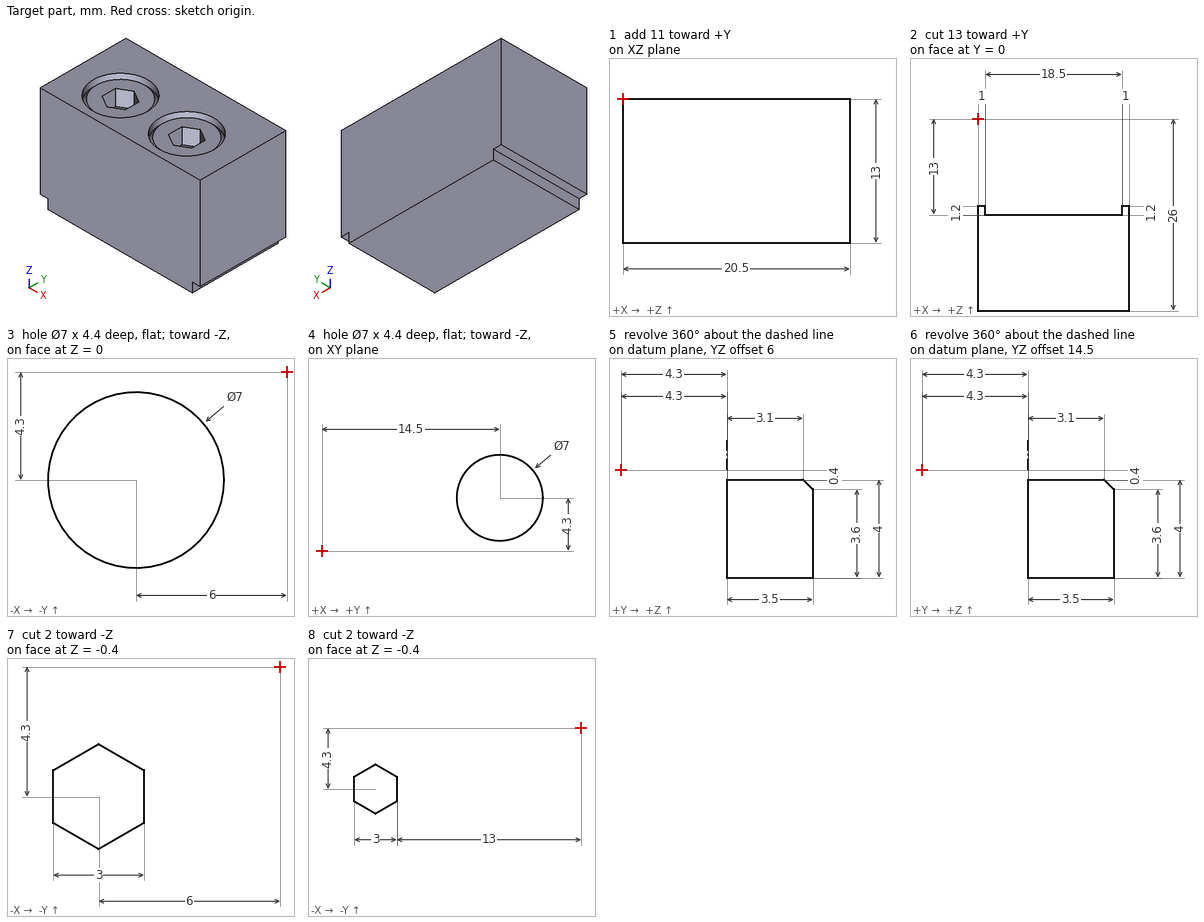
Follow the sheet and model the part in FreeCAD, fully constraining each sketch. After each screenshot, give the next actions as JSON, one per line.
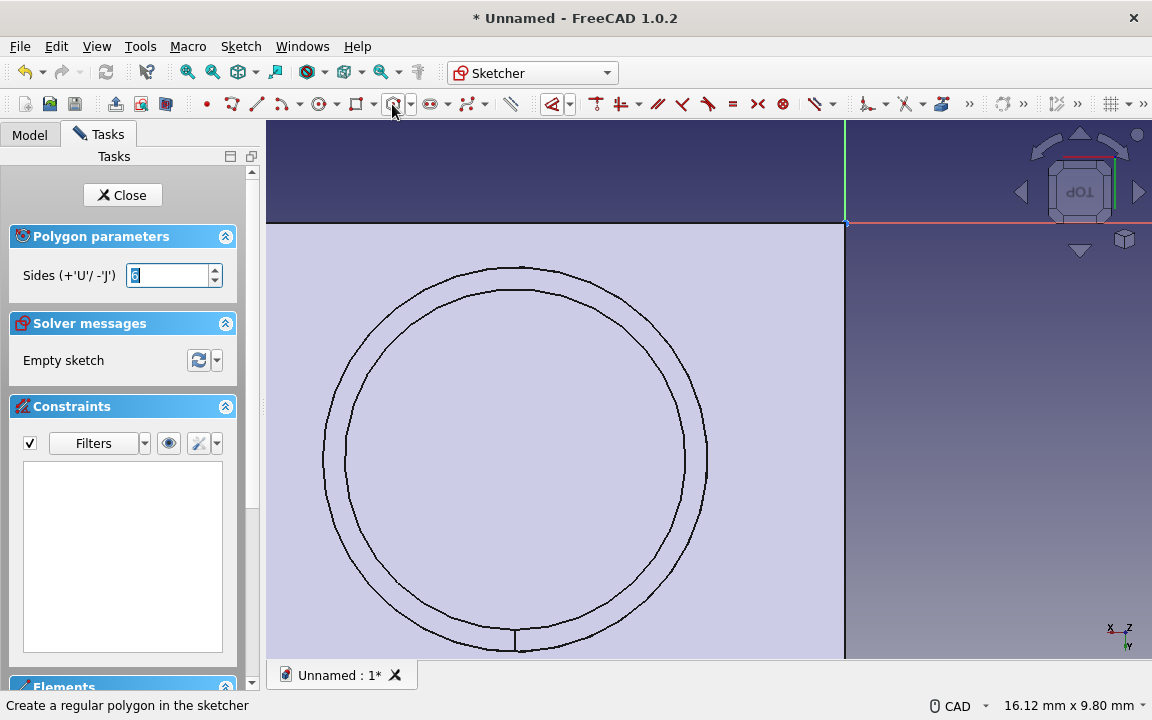
{"action": "left_click", "coordinate": [515, 460]}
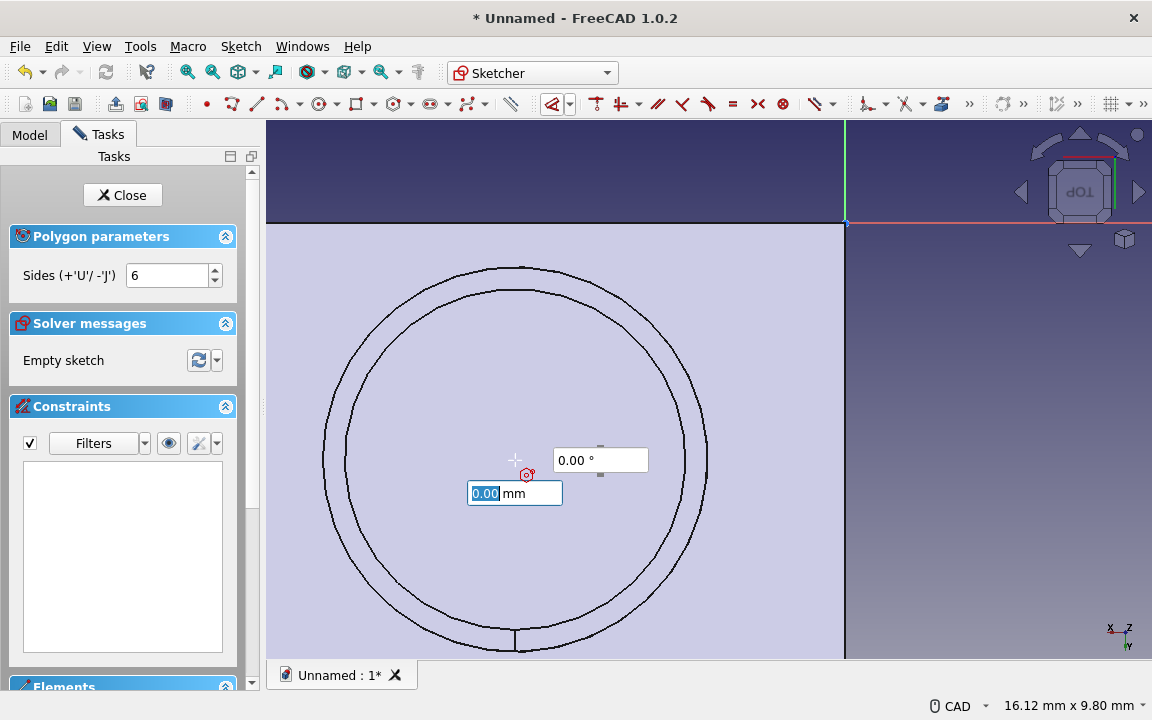
{"action": "left_click", "coordinate": [515, 555]}
{"action": "right_click", "coordinate": [515, 555]}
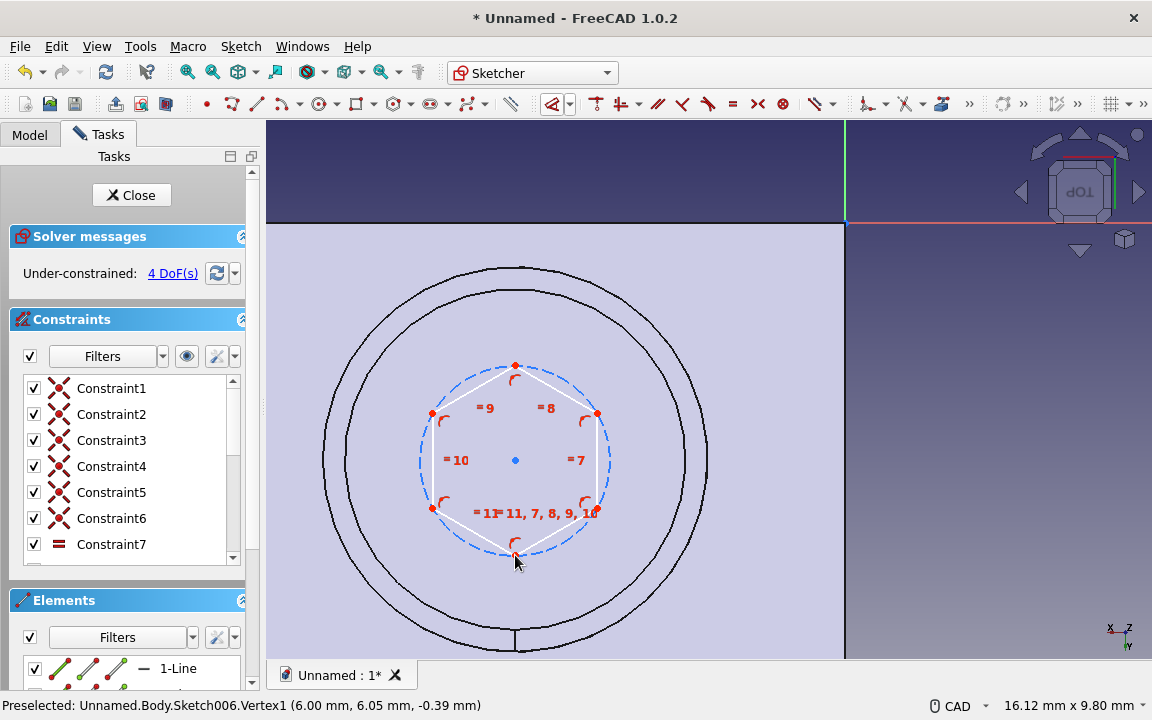
{"action": "scroll", "coordinate": [597, 480], "scroll_direction": "up", "scroll_amount": 2}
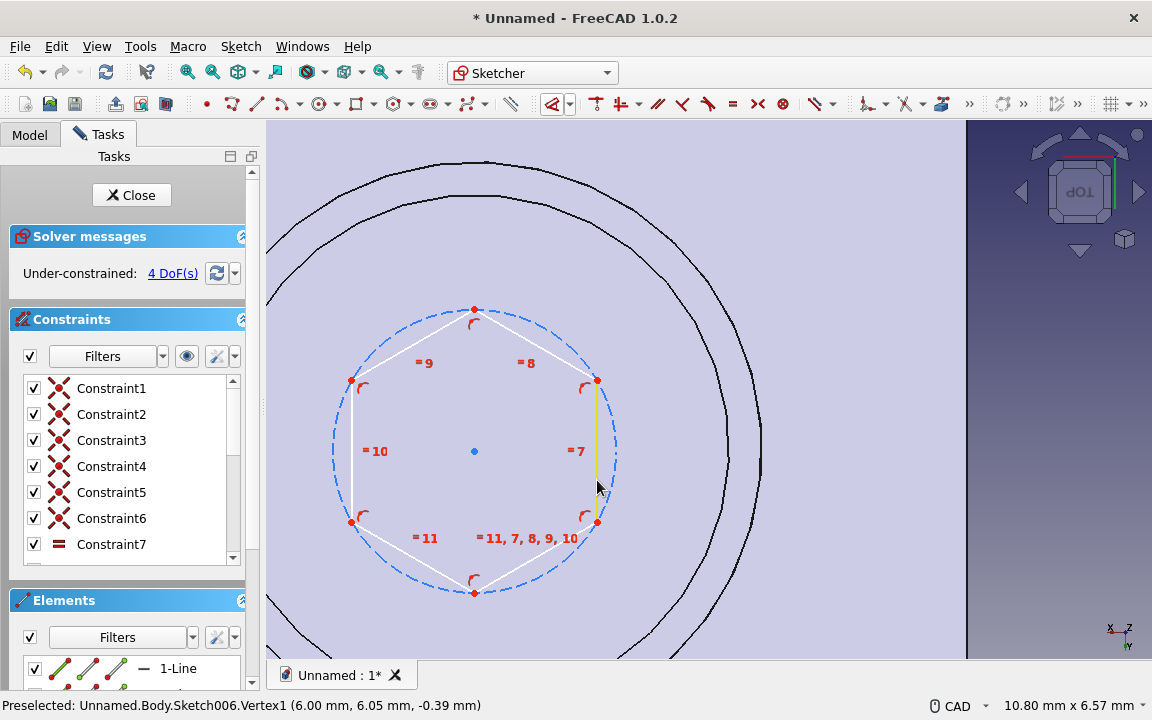
{"action": "left_click", "coordinate": [597, 480]}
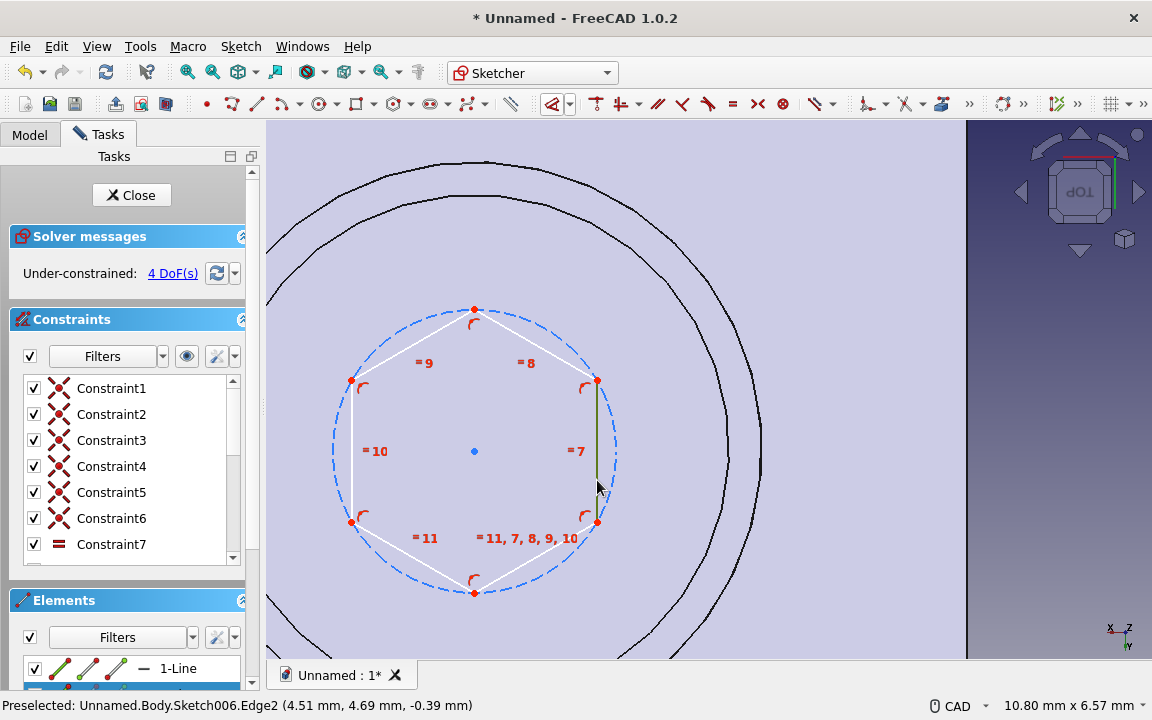
{"action": "left_click", "coordinate": [638, 104]}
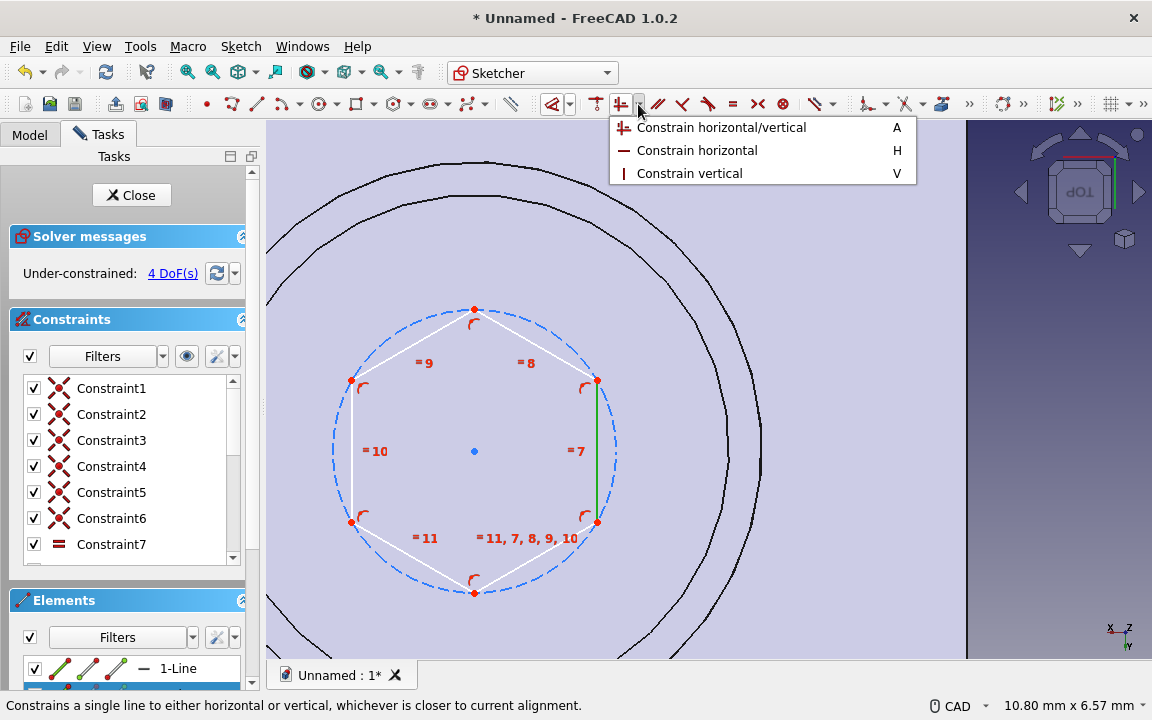
{"action": "left_click", "coordinate": [763, 174]}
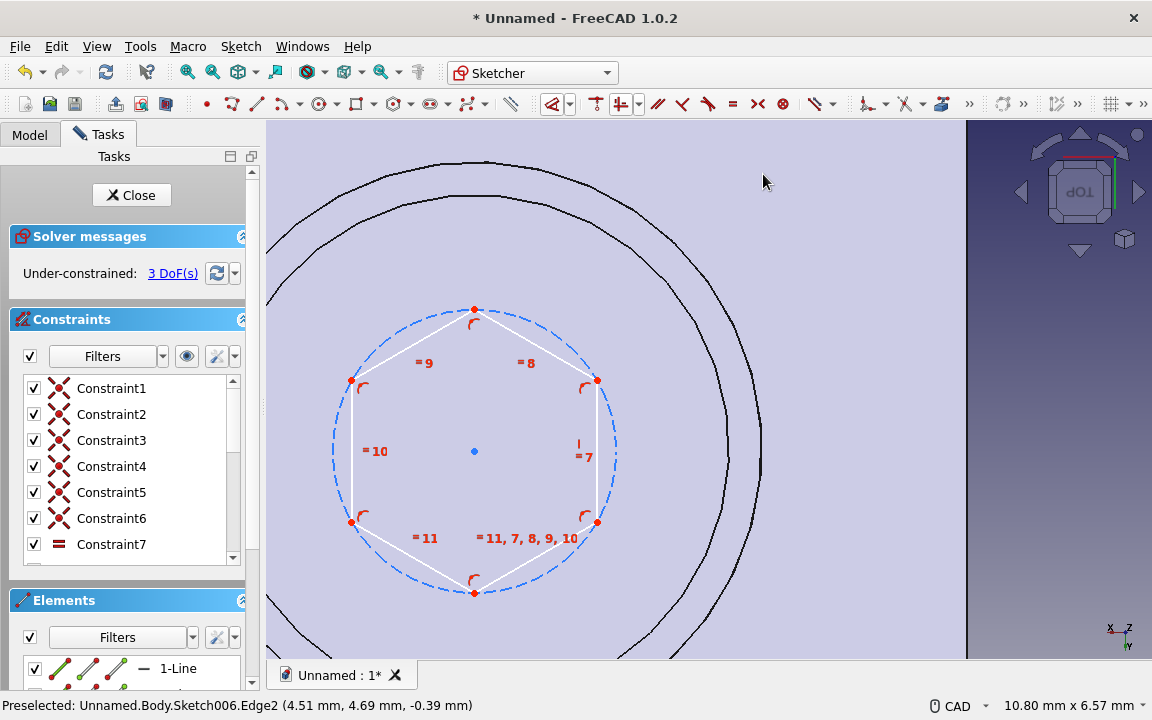
{"action": "left_click", "coordinate": [352, 380]}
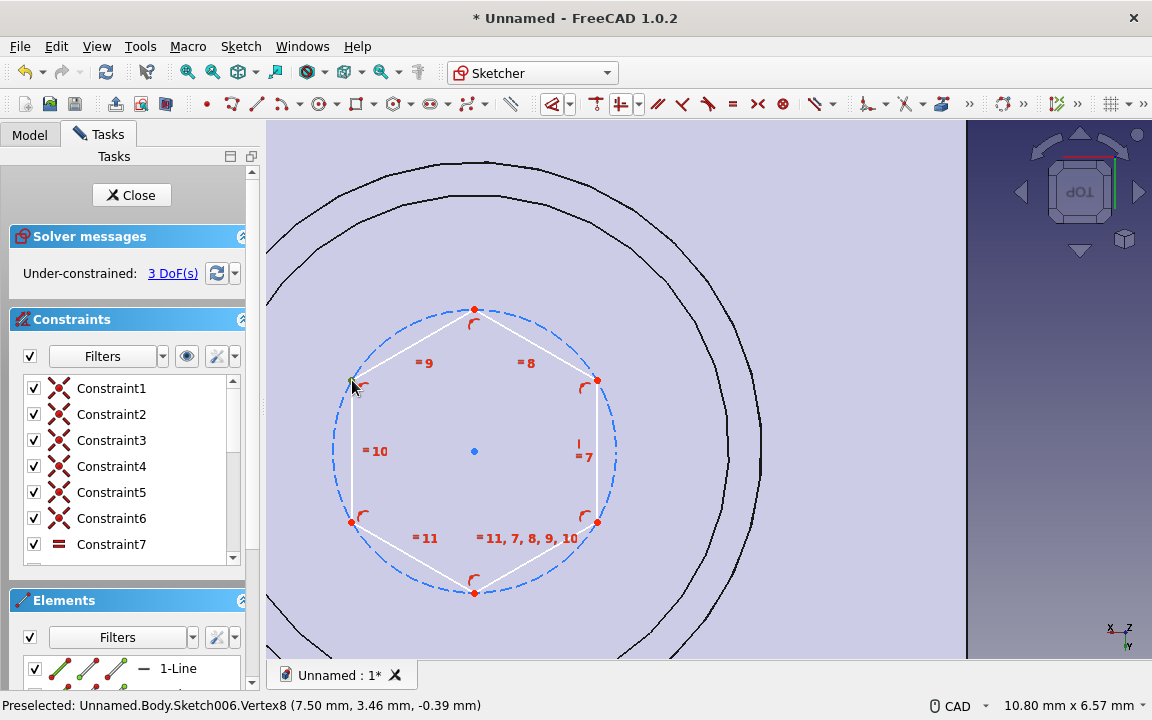
{"action": "left_click", "coordinate": [597, 522]}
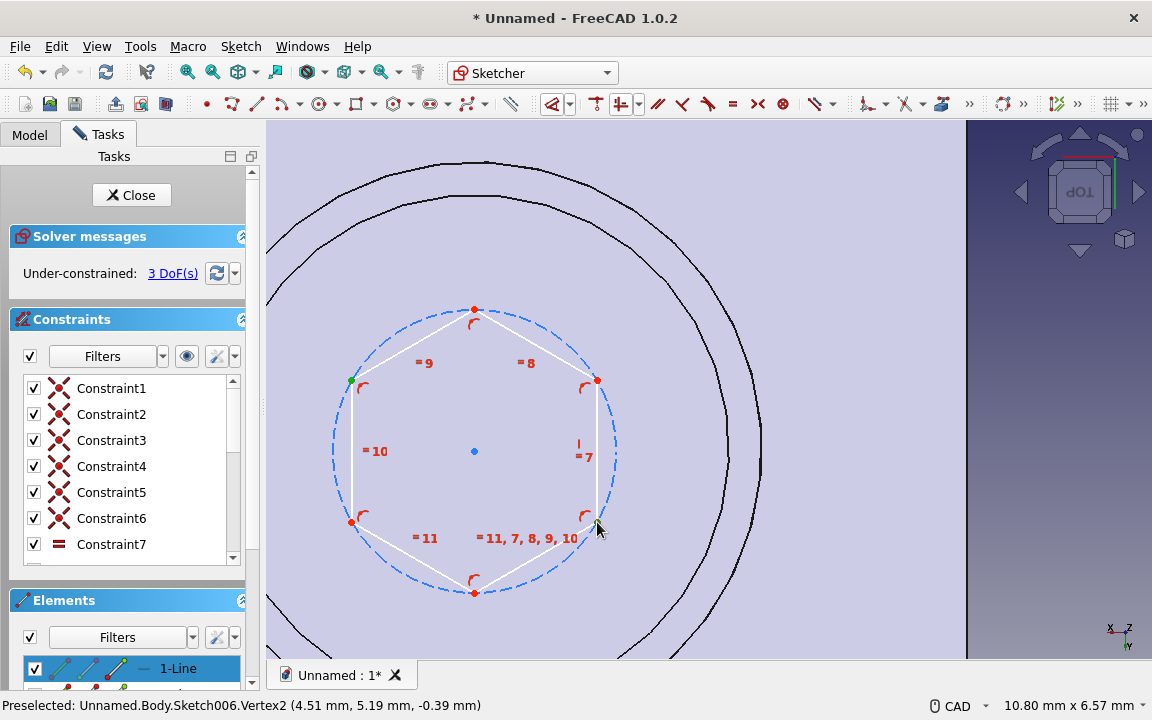
{"action": "key", "text": "l"}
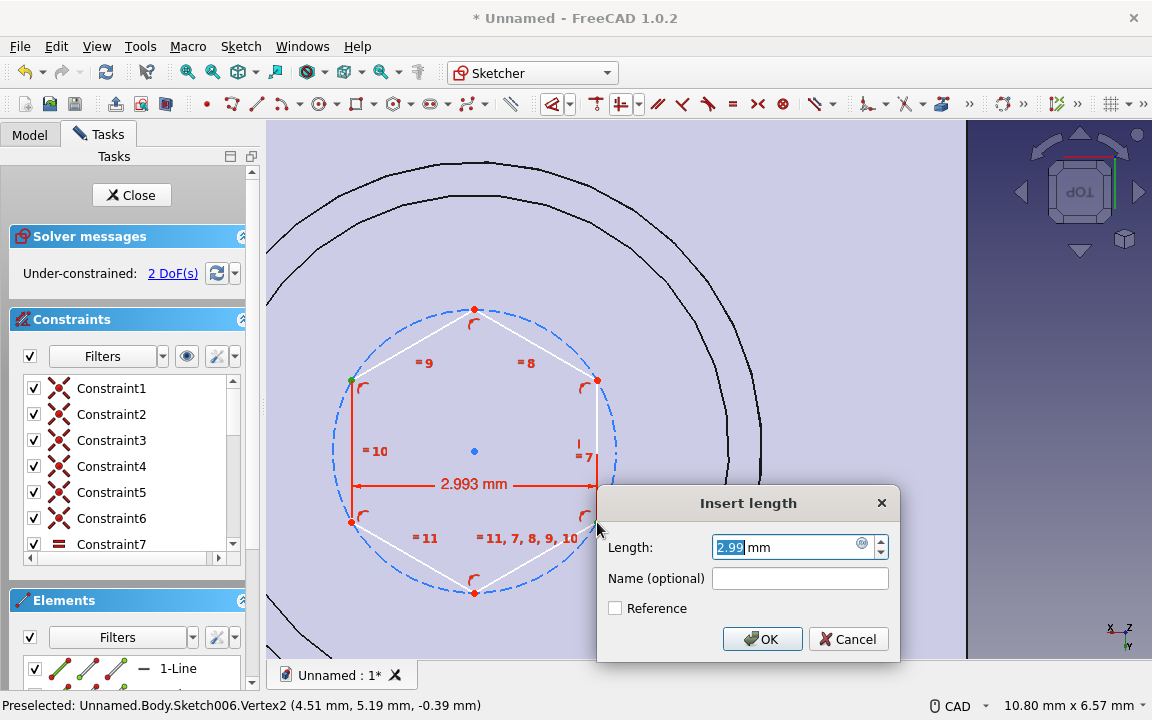
{"action": "type", "text": "3"}
{"action": "key", "text": "Return"}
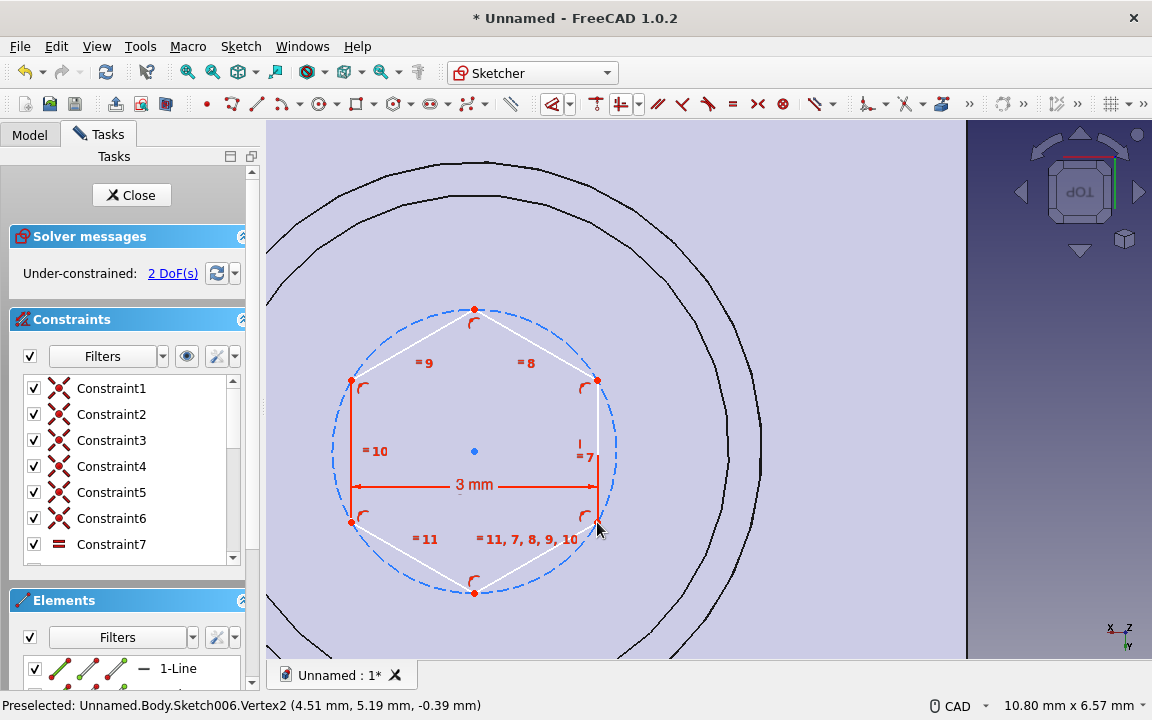
{"action": "left_click", "coordinate": [474, 451]}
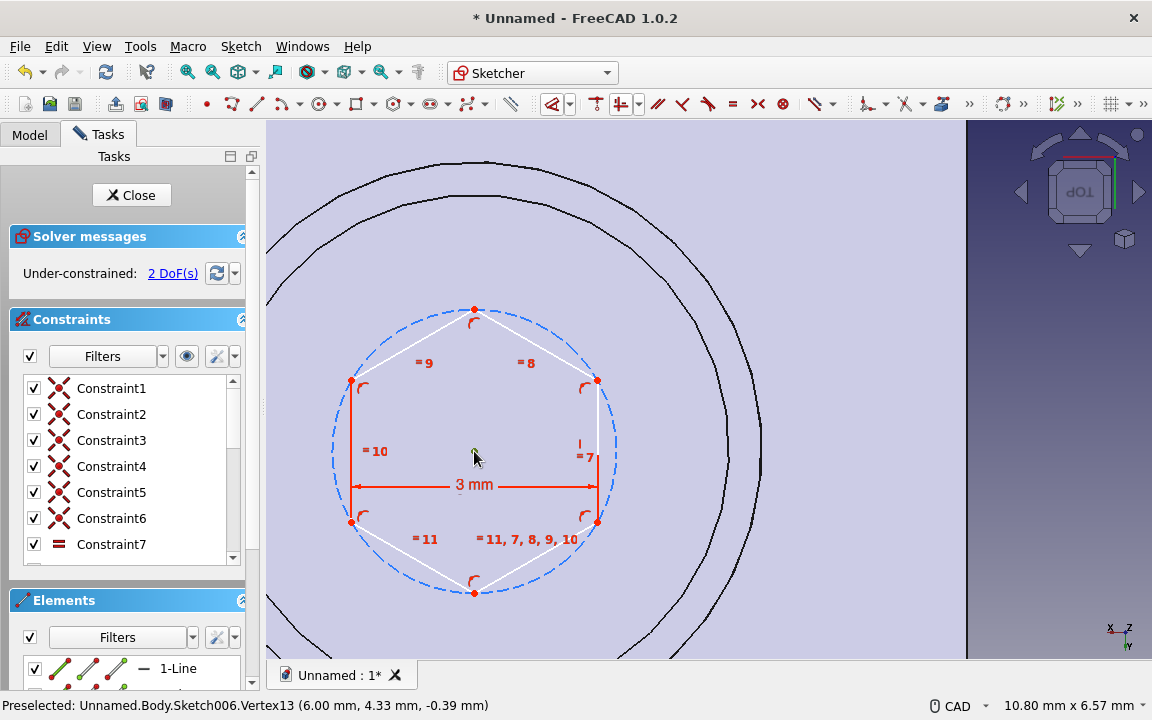
{"action": "left_click", "coordinate": [570, 104]}